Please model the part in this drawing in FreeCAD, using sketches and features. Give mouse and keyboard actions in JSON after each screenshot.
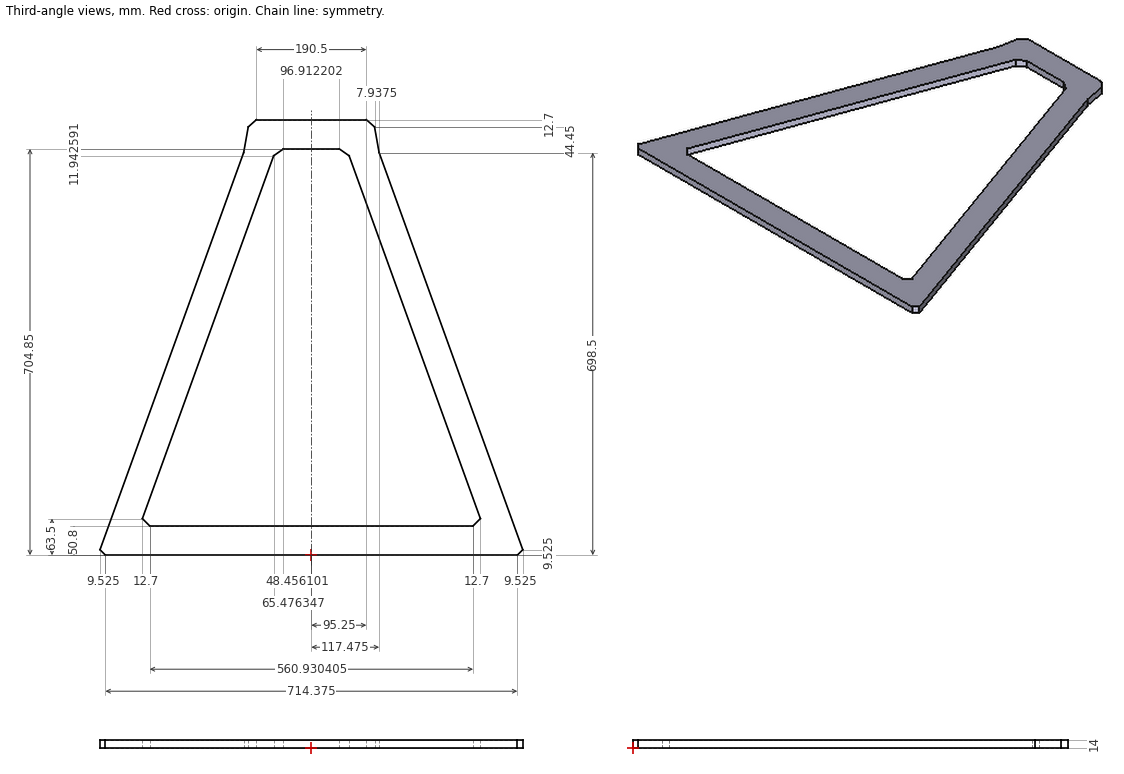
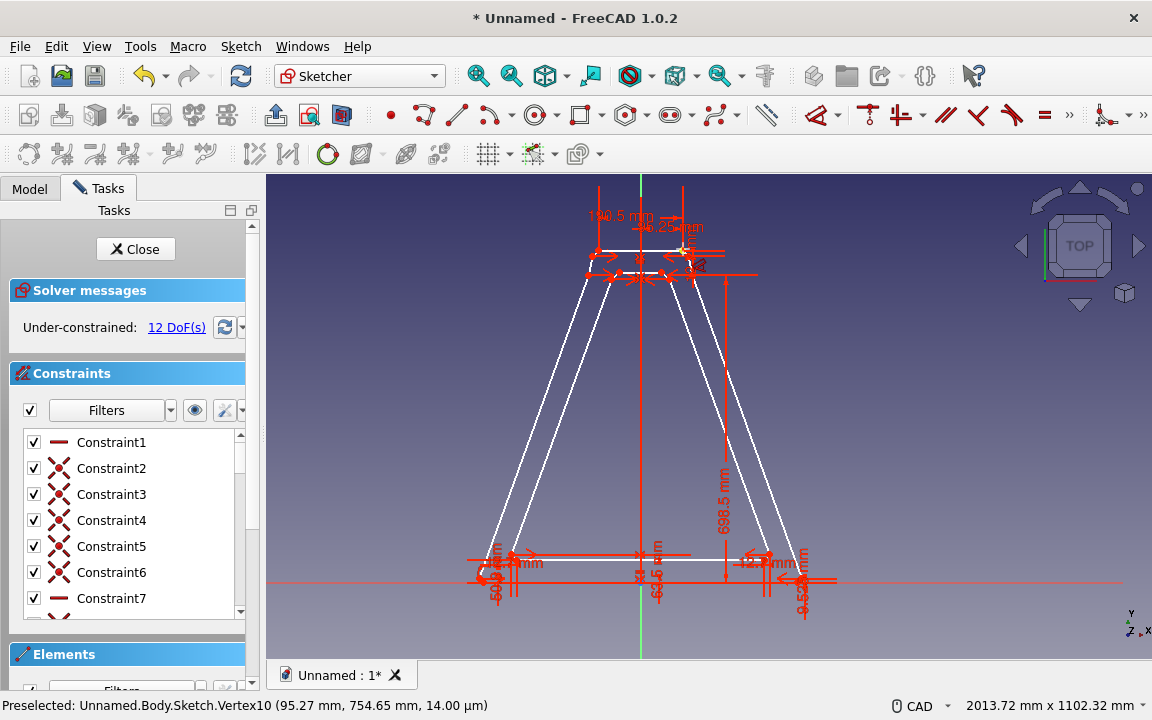
{"action": "scroll", "coordinate": [800, 581], "scroll_direction": "up", "scroll_amount": 12}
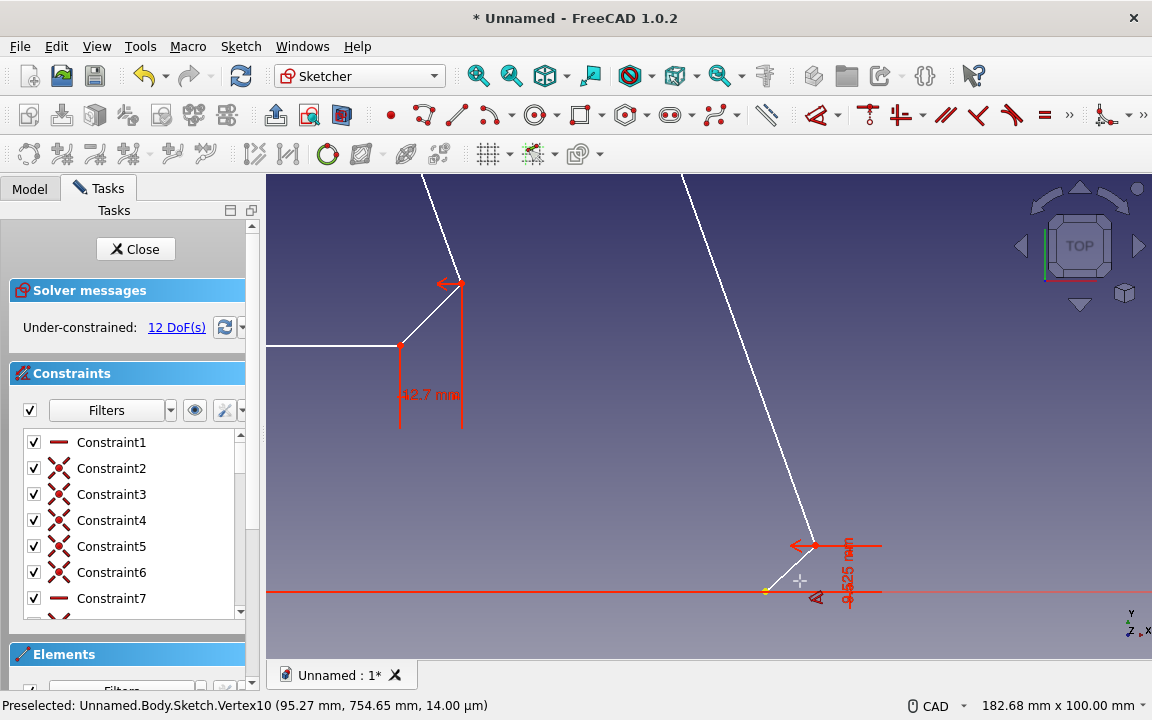
{"action": "left_click", "coordinate": [791, 569]}
{"action": "left_click", "coordinate": [791, 626]}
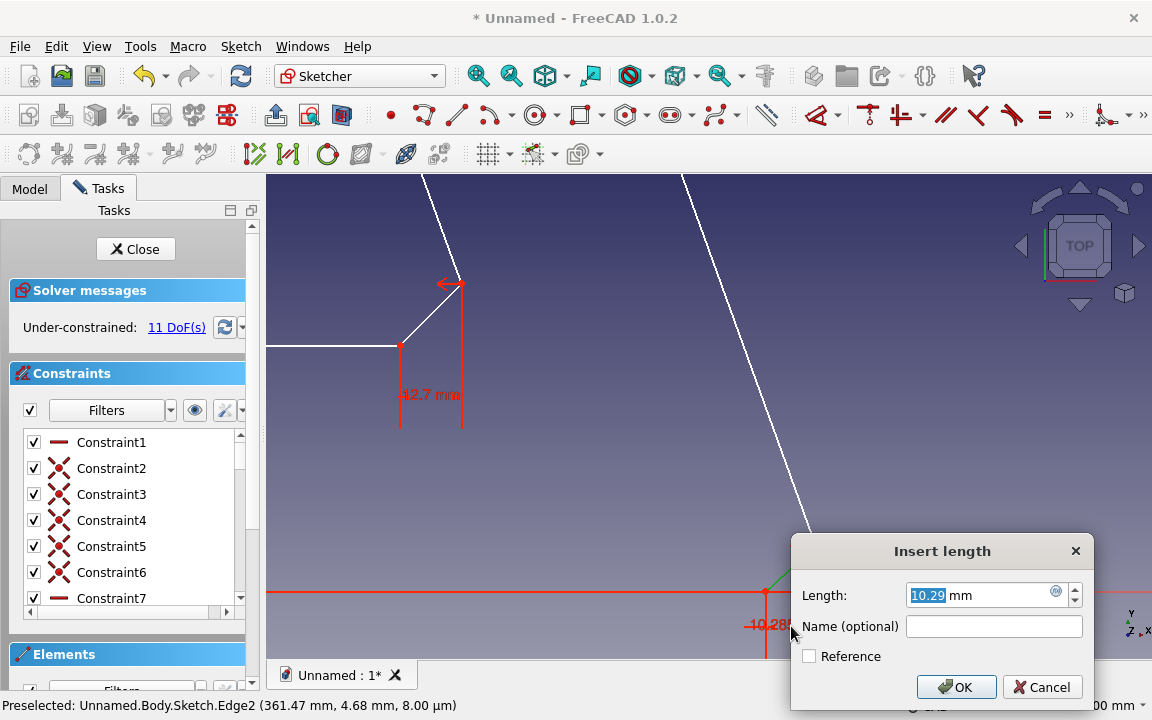
{"action": "type", "text": "9.525"}
{"action": "key", "text": "Return"}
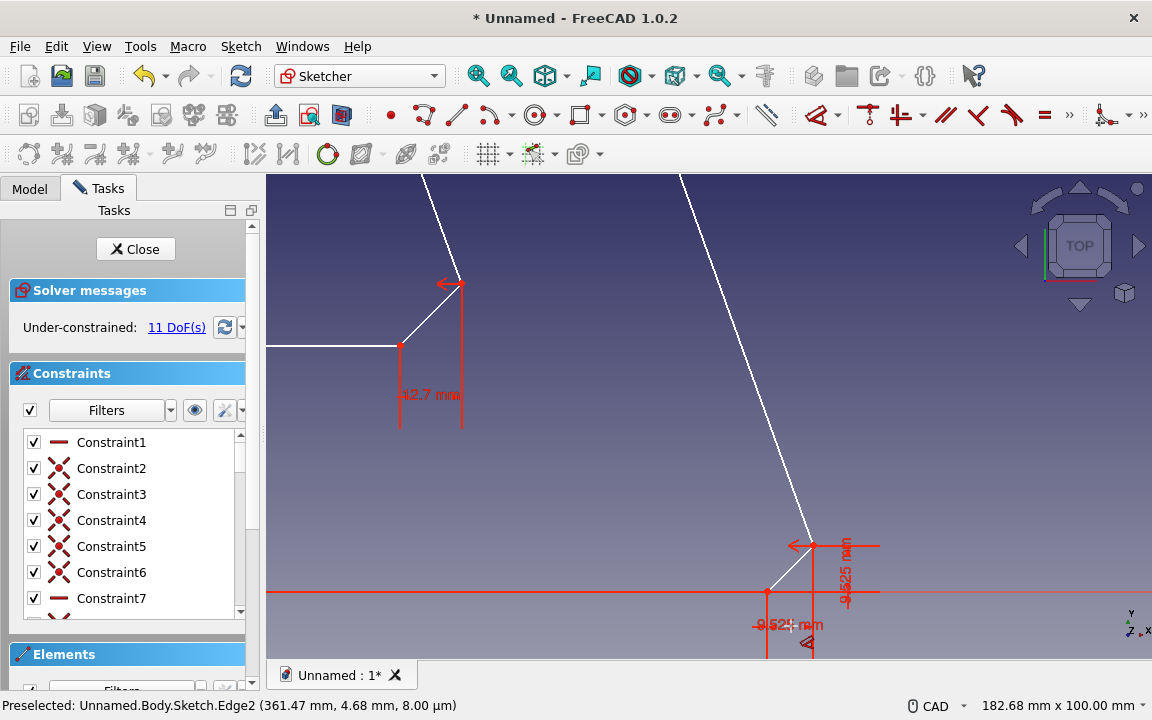
{"action": "scroll", "coordinate": [800, 582], "scroll_direction": "down", "scroll_amount": 12}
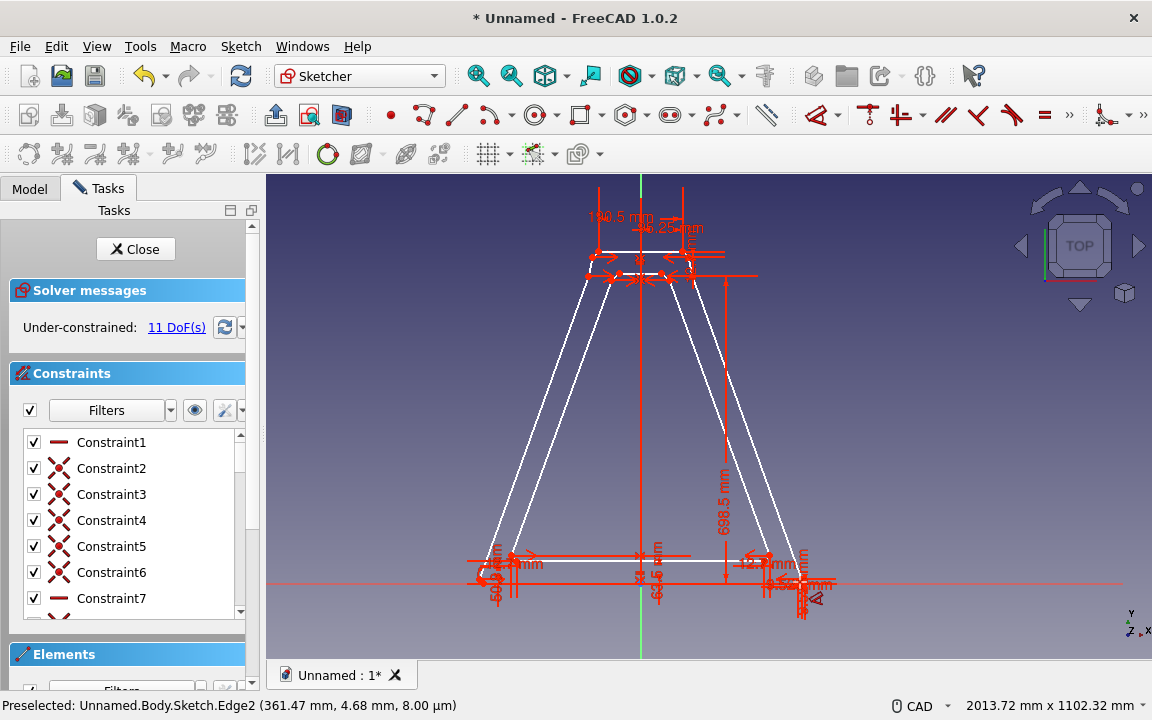
{"action": "scroll", "coordinate": [691, 271], "scroll_direction": "up", "scroll_amount": 5}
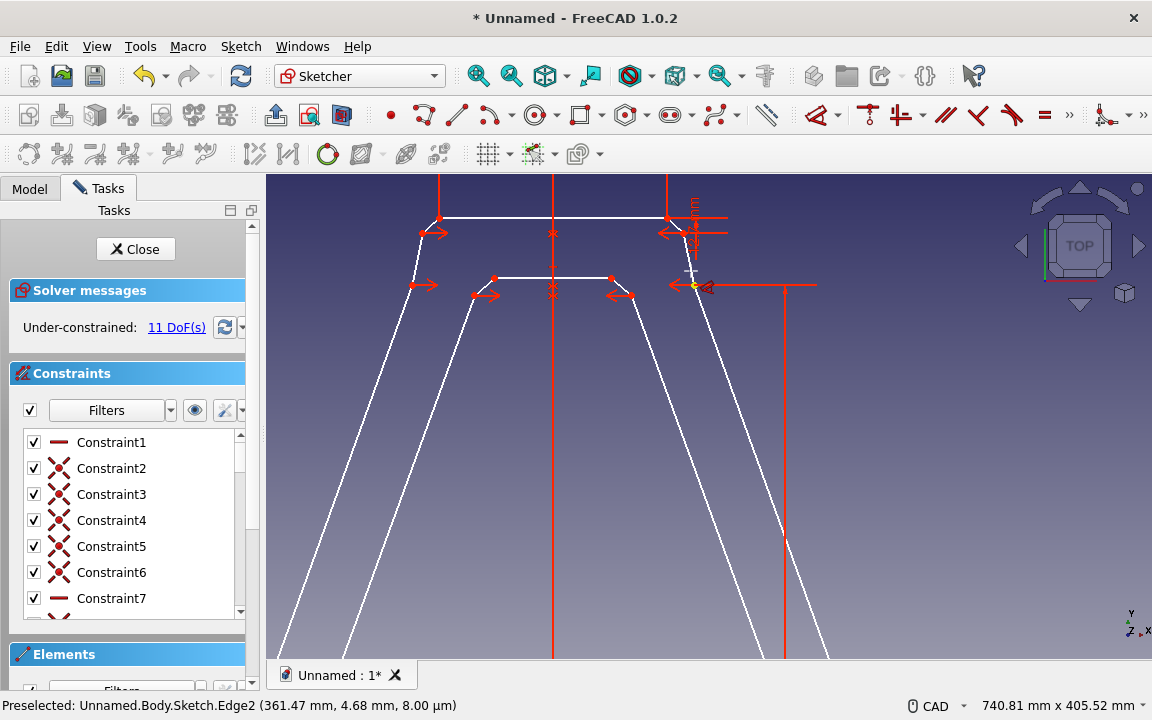
{"action": "left_click", "coordinate": [691, 270]}
{"action": "left_click", "coordinate": [728, 259]}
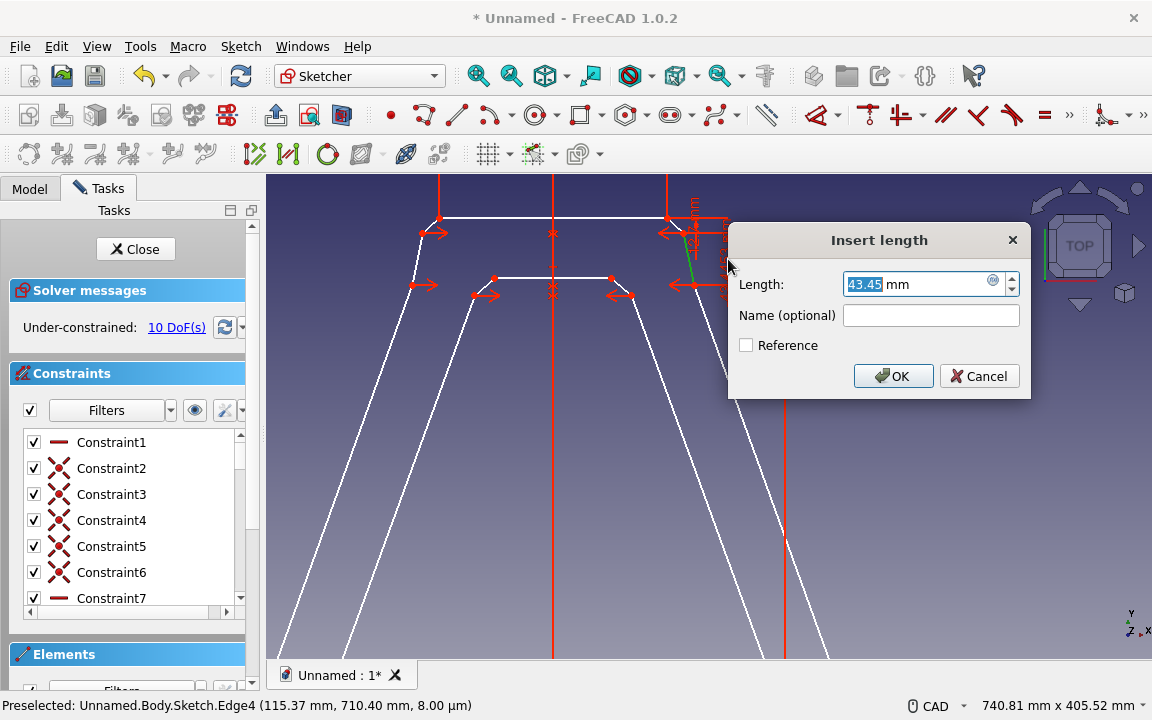
{"action": "type", "text": "44.45"}
{"action": "key", "text": "Return"}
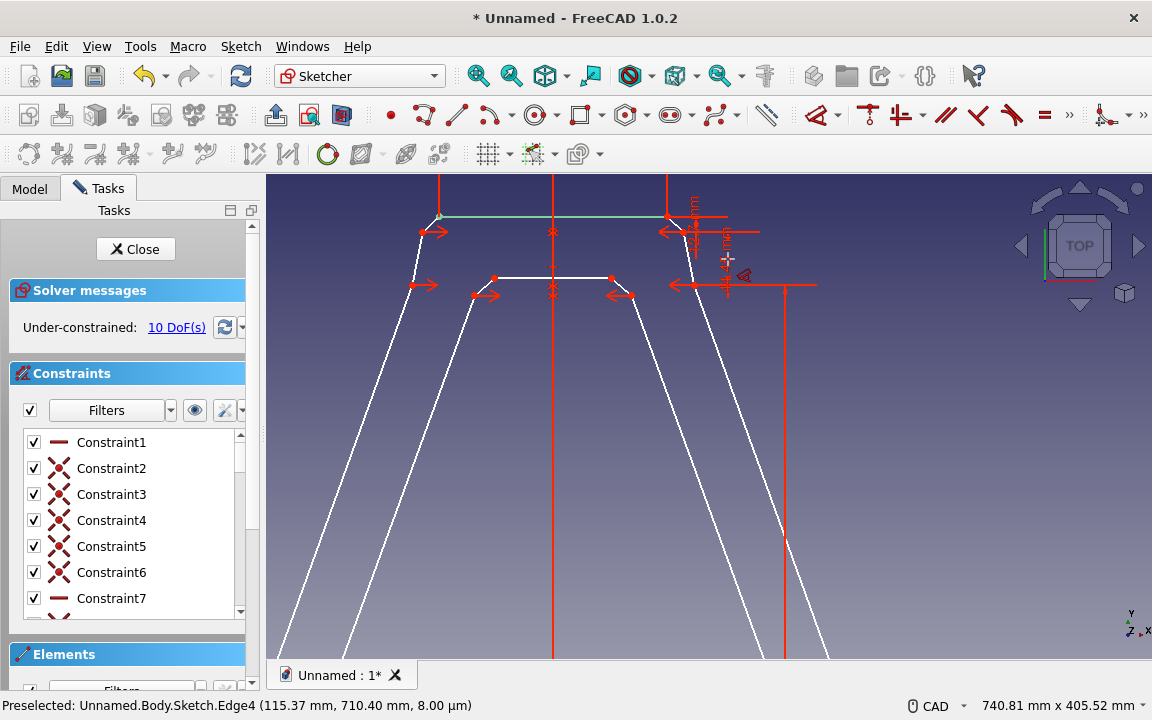
{"action": "scroll", "coordinate": [691, 270], "scroll_direction": "down", "scroll_amount": 5}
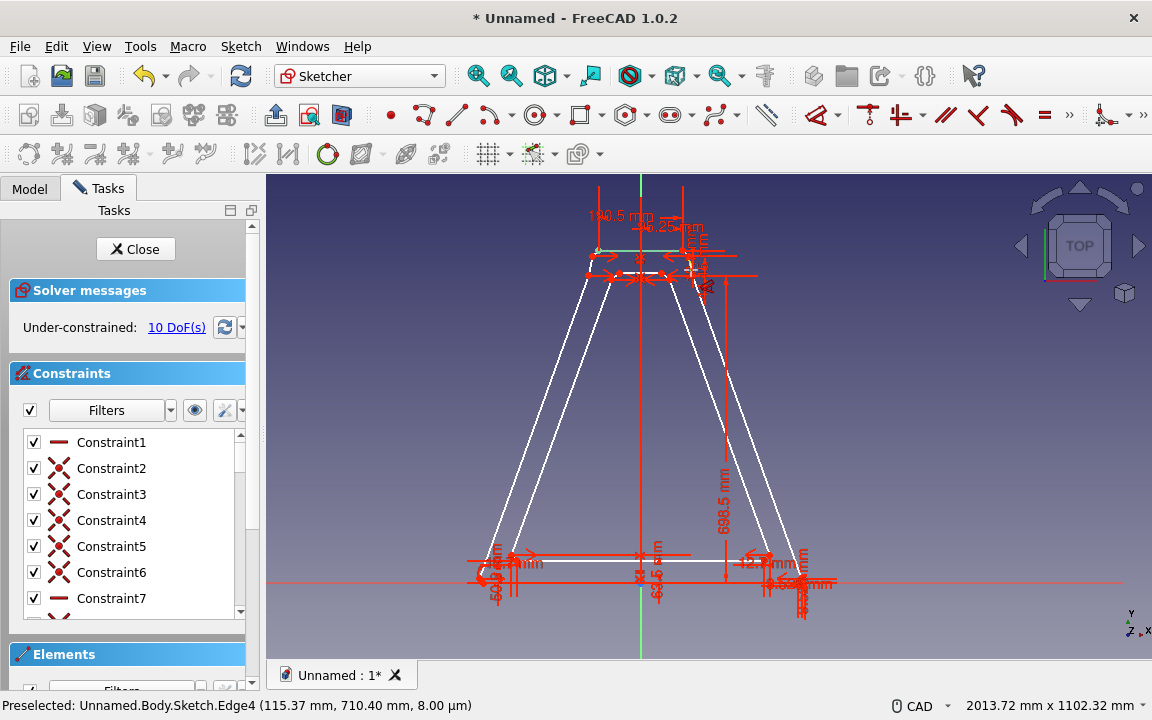
{"action": "scroll", "coordinate": [481, 581], "scroll_direction": "up", "scroll_amount": 12}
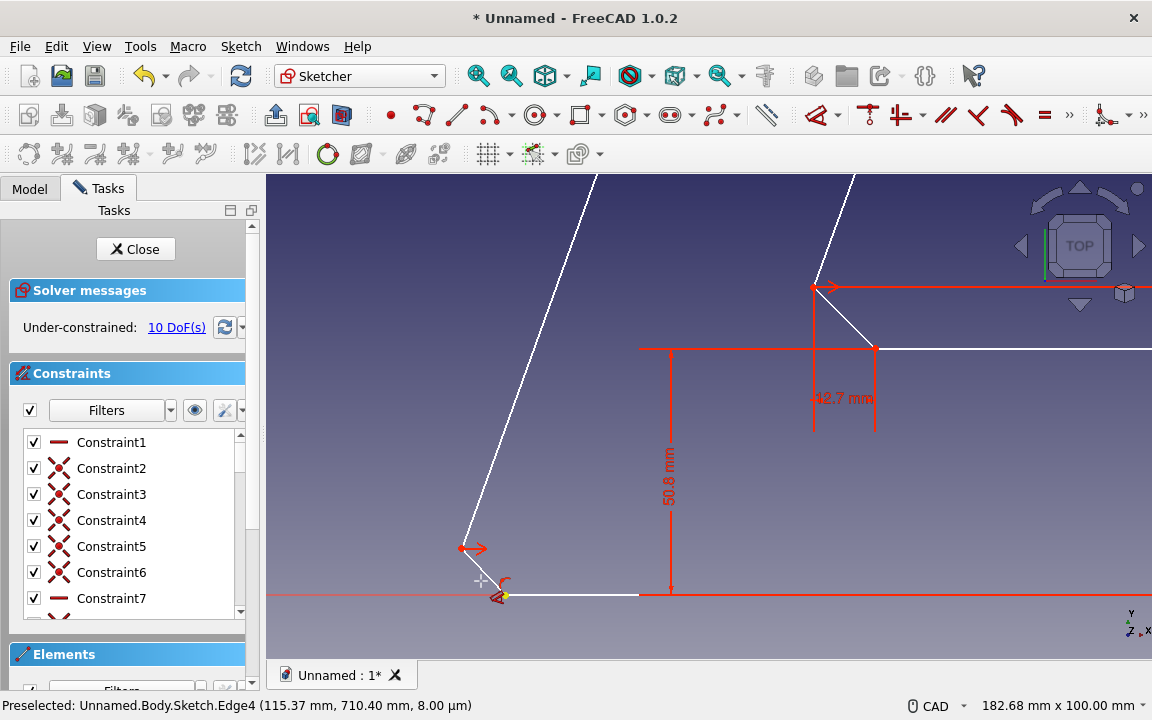
{"action": "left_click", "coordinate": [479, 567]}
{"action": "left_click", "coordinate": [484, 629]}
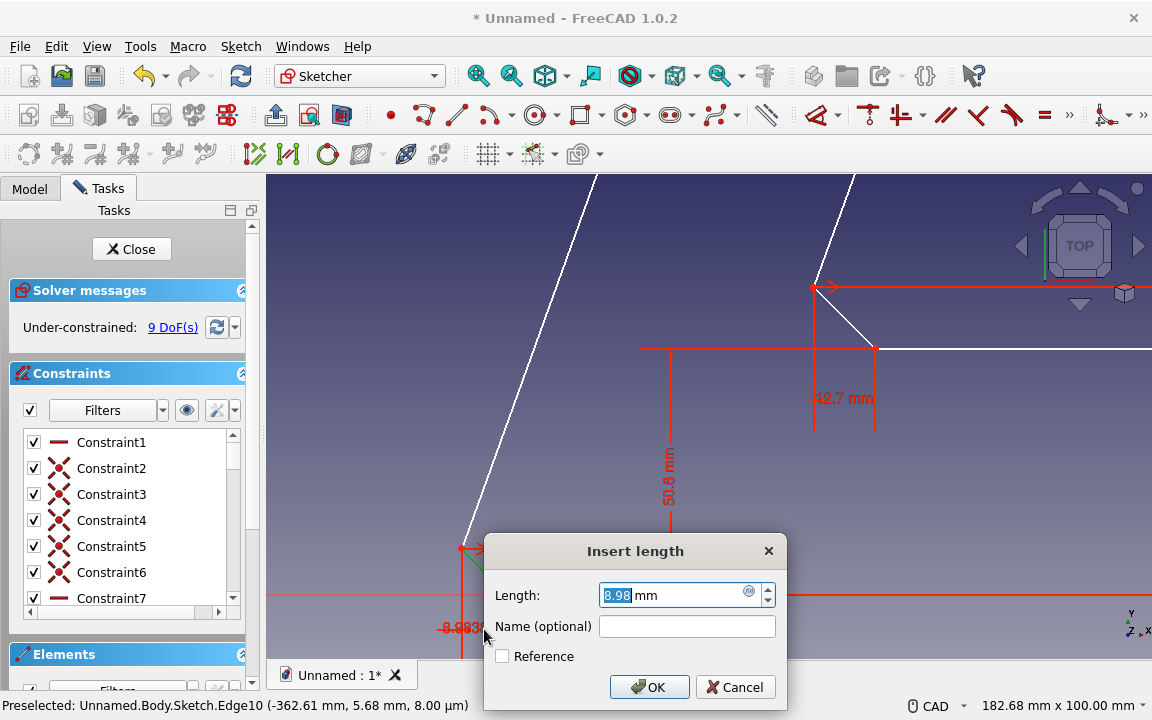
{"action": "type", "text": "9.525"}
{"action": "key", "text": "Return"}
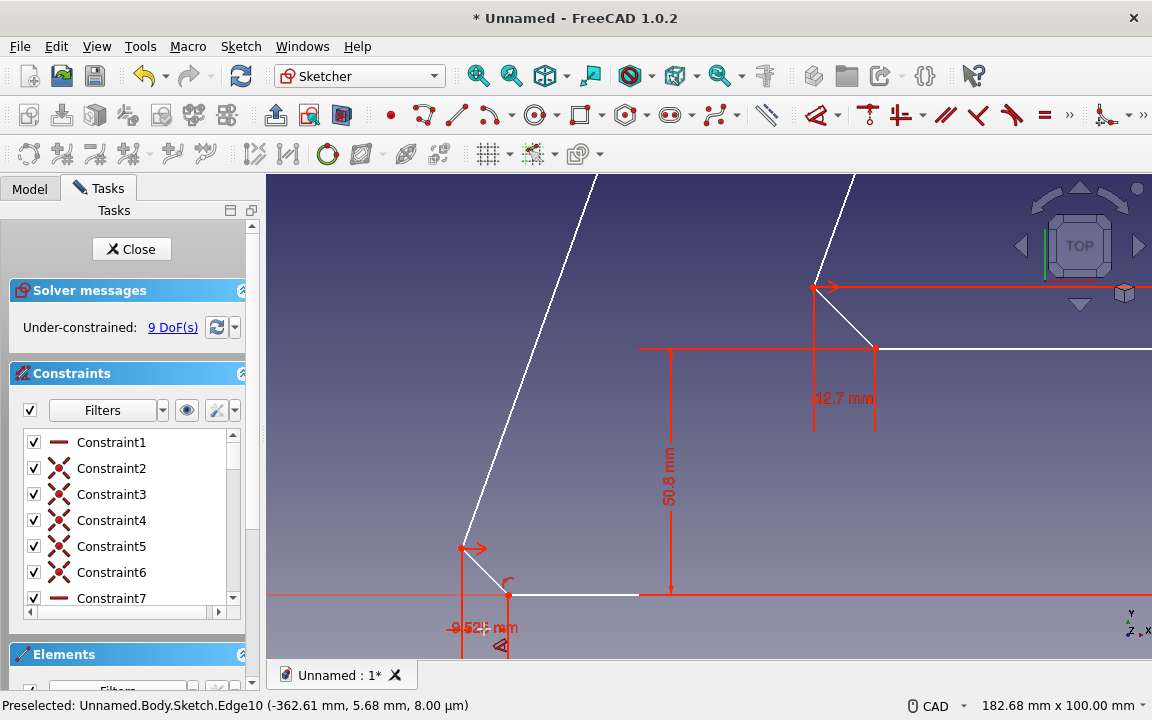
{"action": "scroll", "coordinate": [481, 582], "scroll_direction": "down", "scroll_amount": 12}